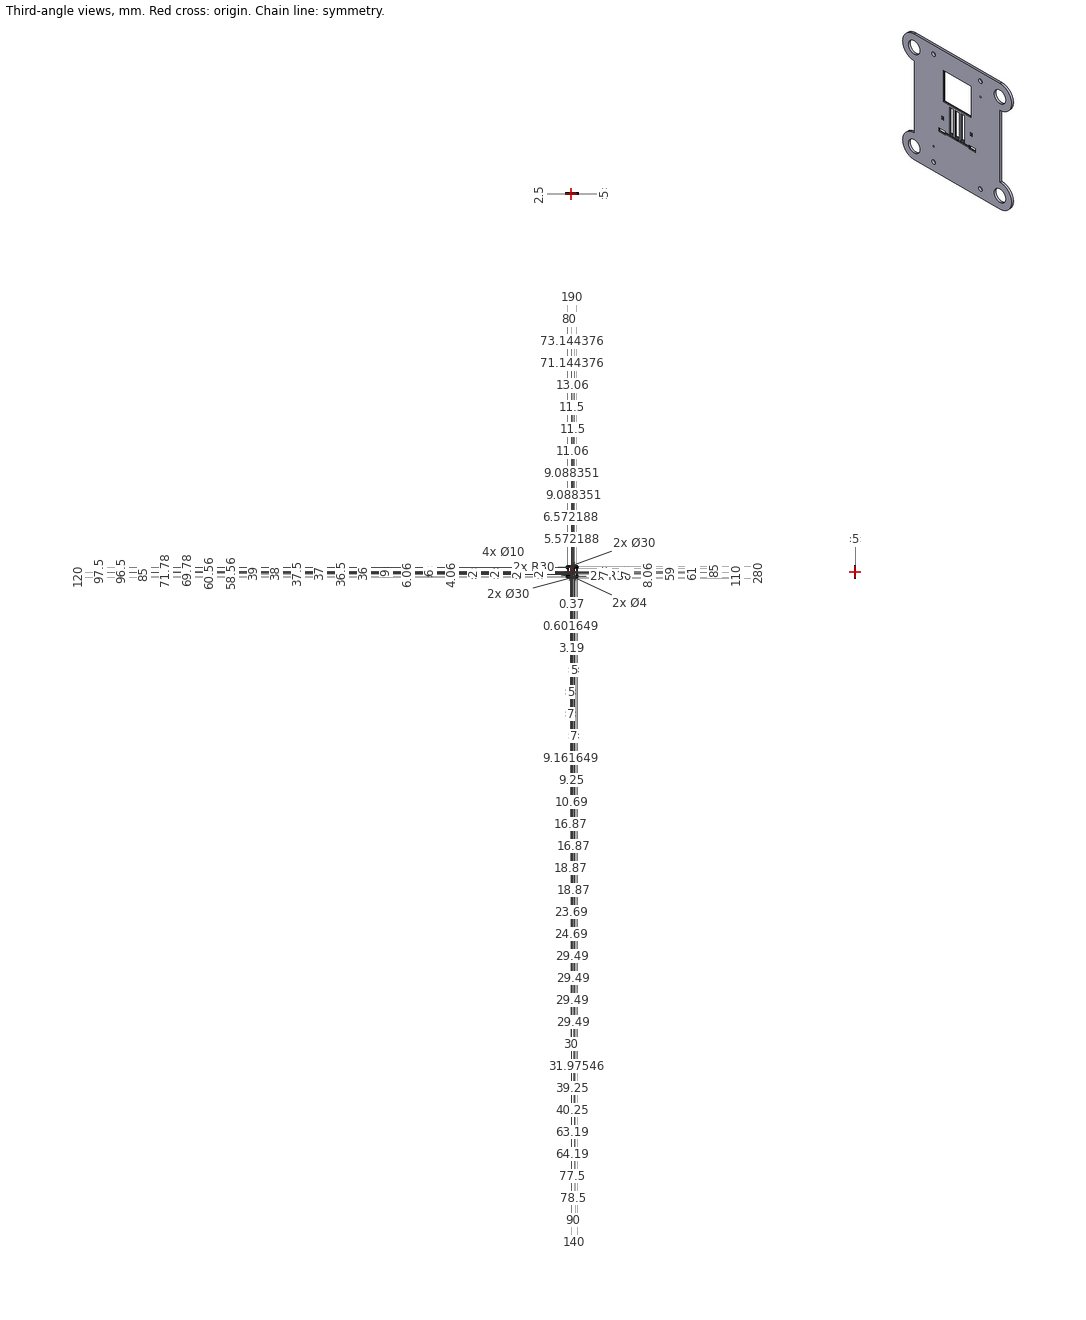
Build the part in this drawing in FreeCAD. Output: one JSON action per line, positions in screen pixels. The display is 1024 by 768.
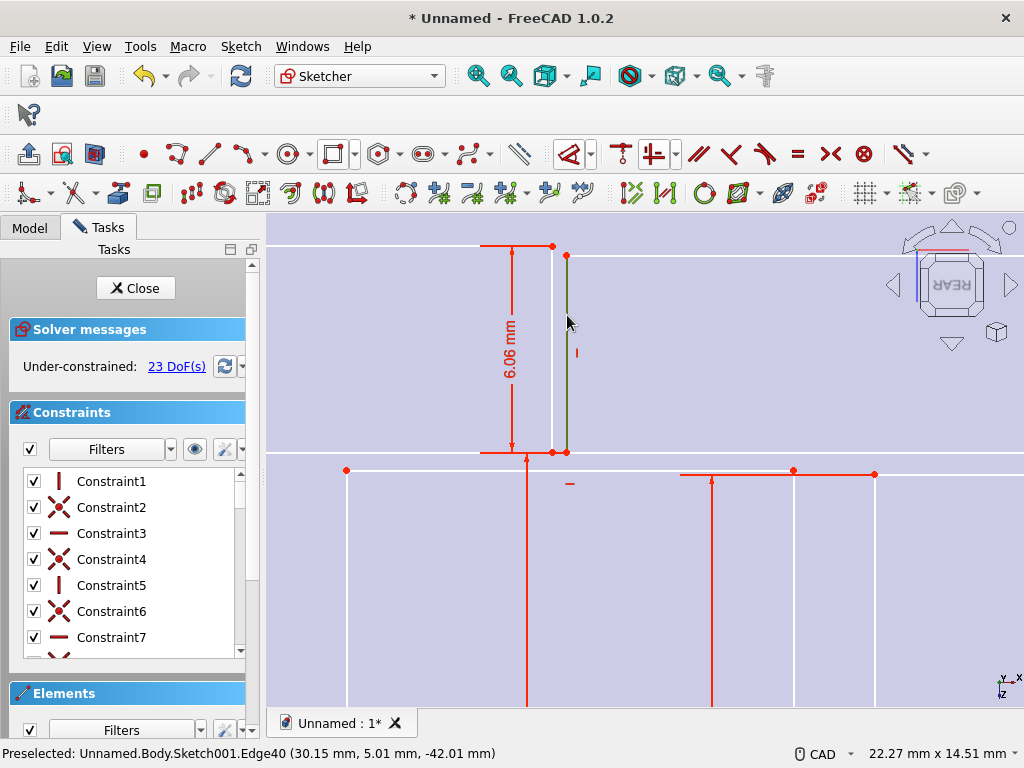
{"action": "left_click", "coordinate": [590, 154]}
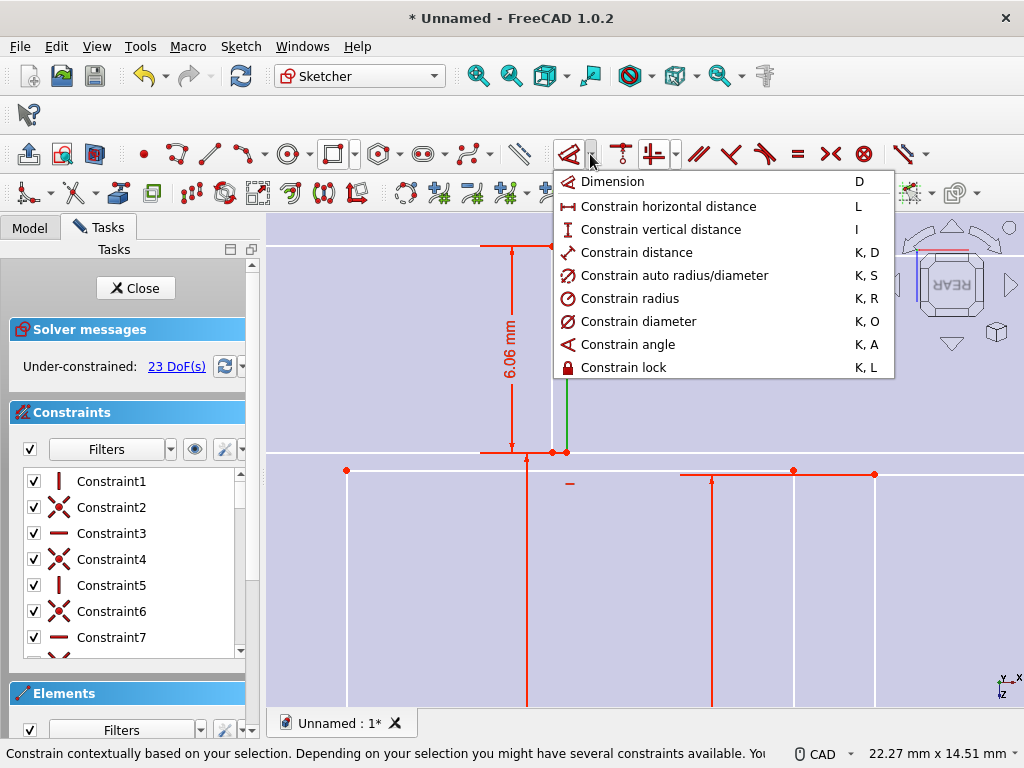
{"action": "left_click", "coordinate": [724, 230]}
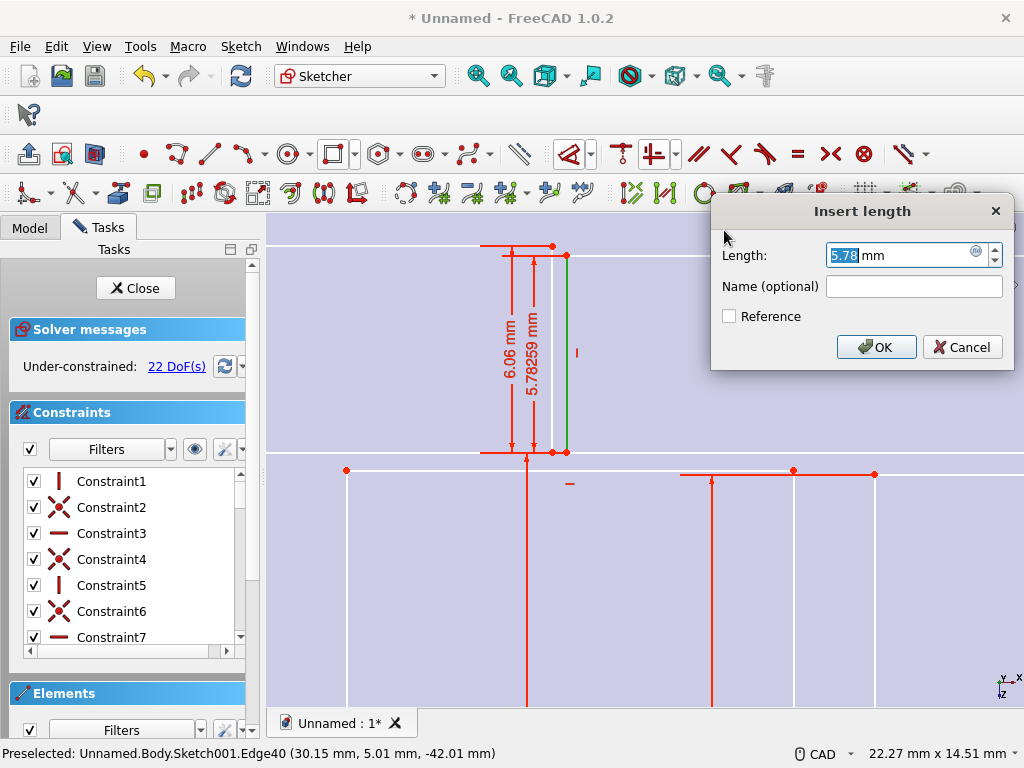
{"action": "type", "text": "6.06"}
{"action": "key", "text": "Return"}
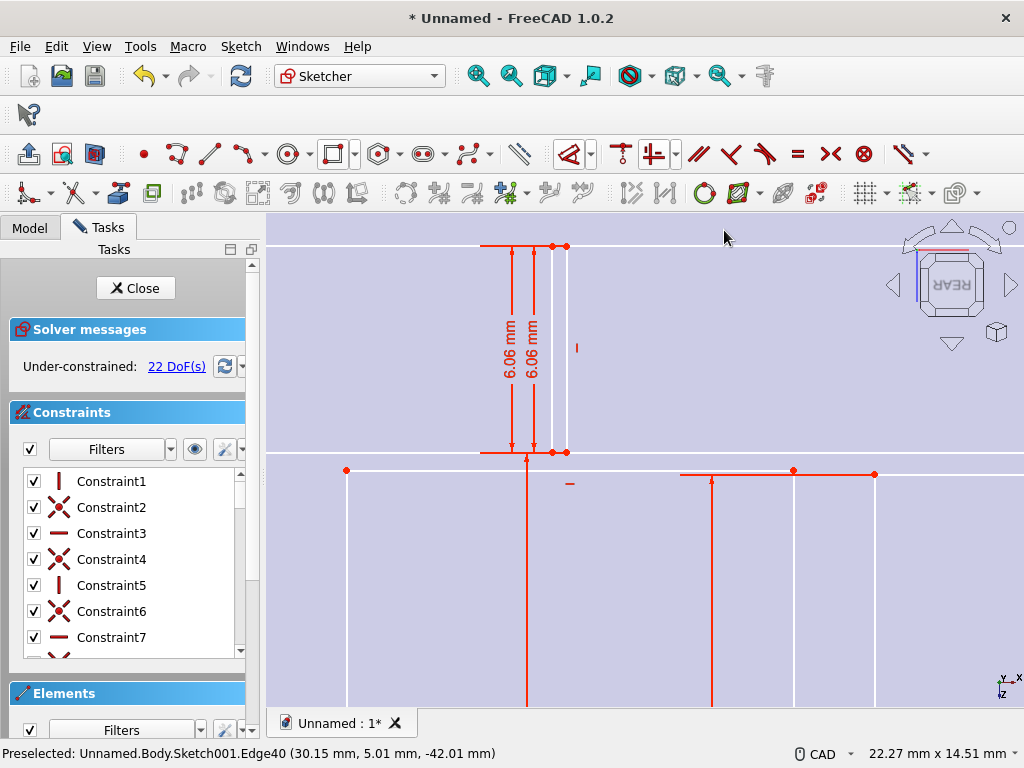
{"action": "left_click", "coordinate": [353, 452]}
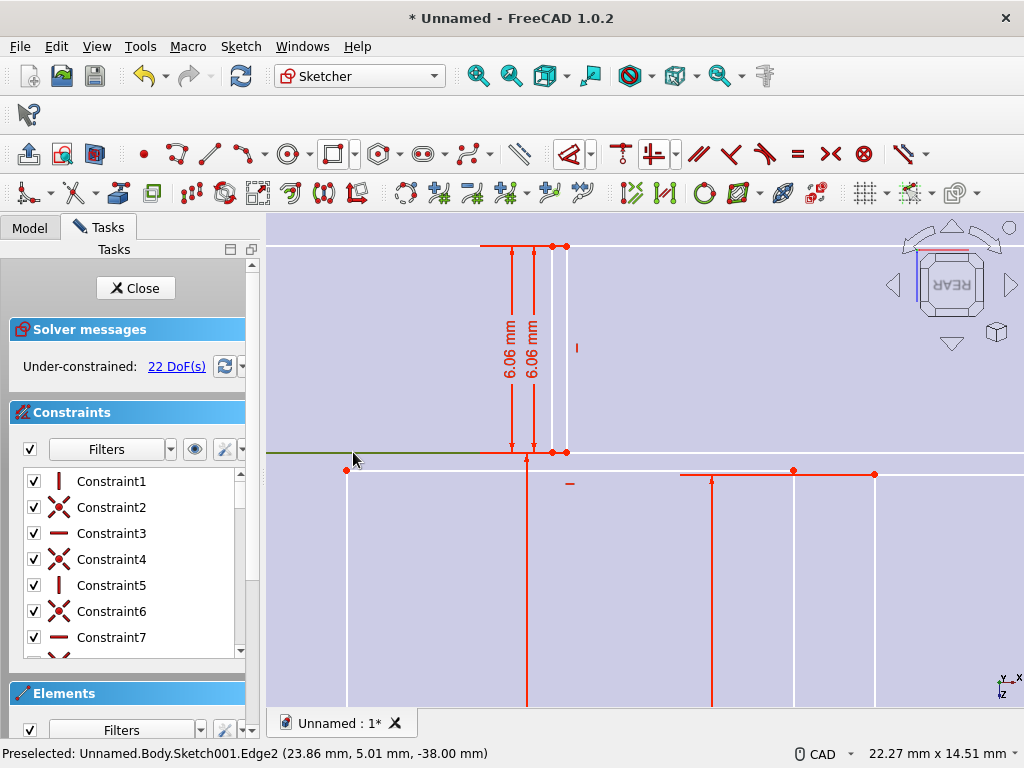
{"action": "left_click", "coordinate": [590, 154]}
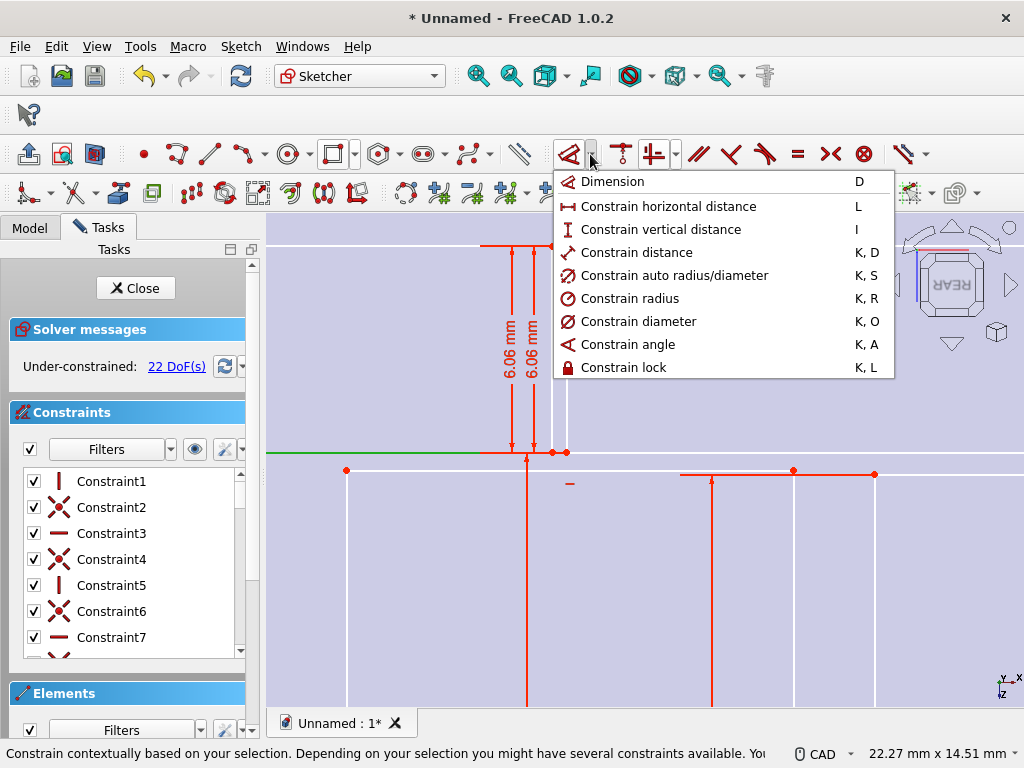
{"action": "left_click", "coordinate": [724, 206]}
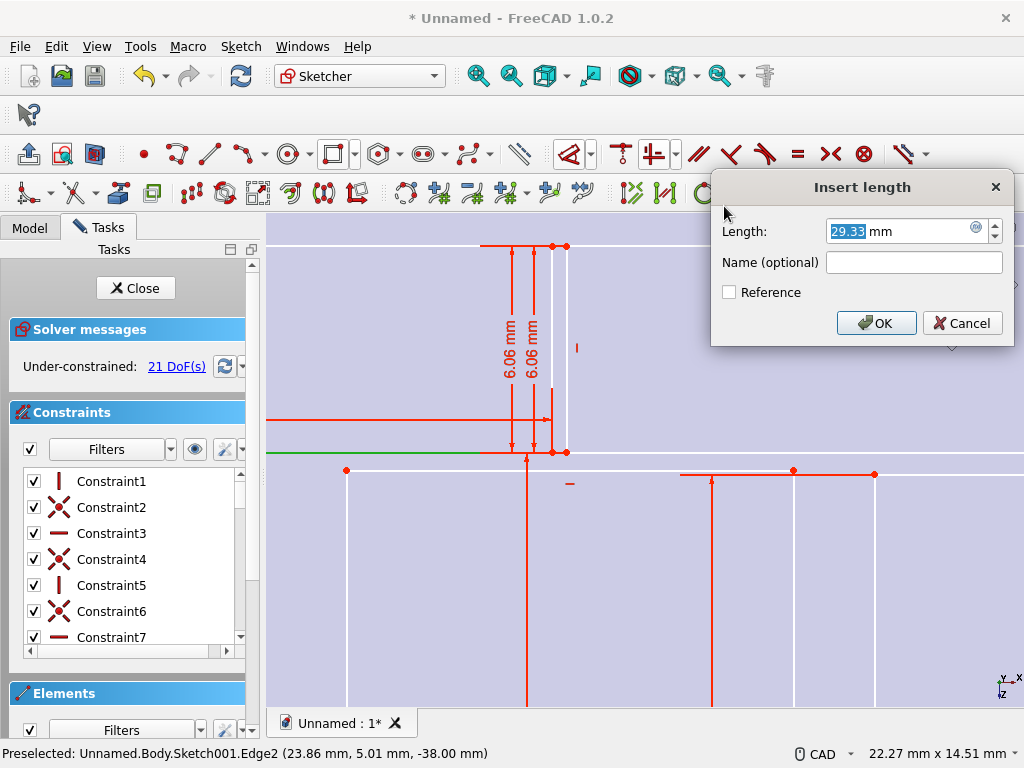
{"action": "type", "text": "29.49"}
{"action": "key", "text": "Return"}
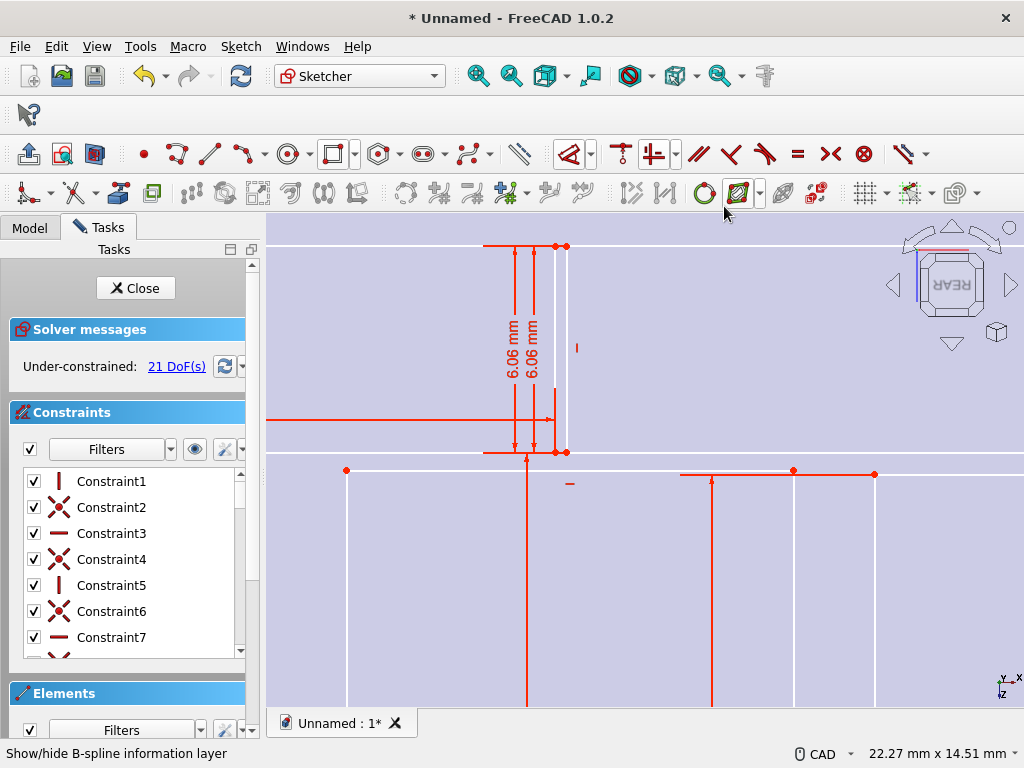
{"action": "scroll", "coordinate": [577, 320], "scroll_direction": "down", "scroll_amount": 14}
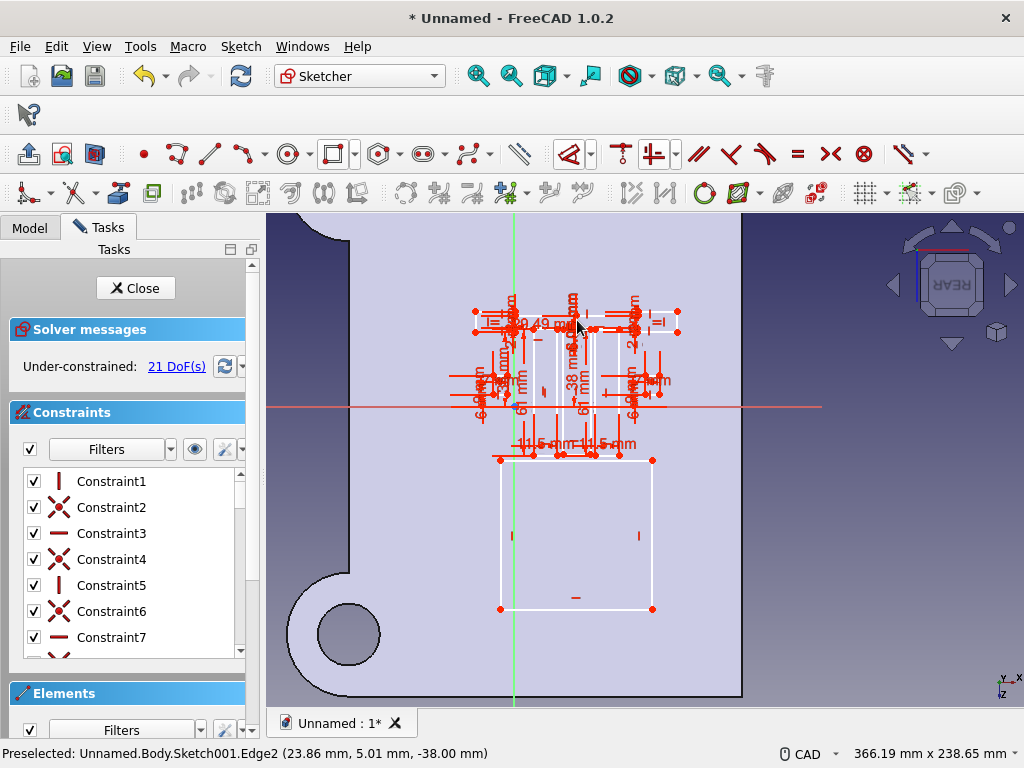
{"action": "left_click", "coordinate": [564, 316]}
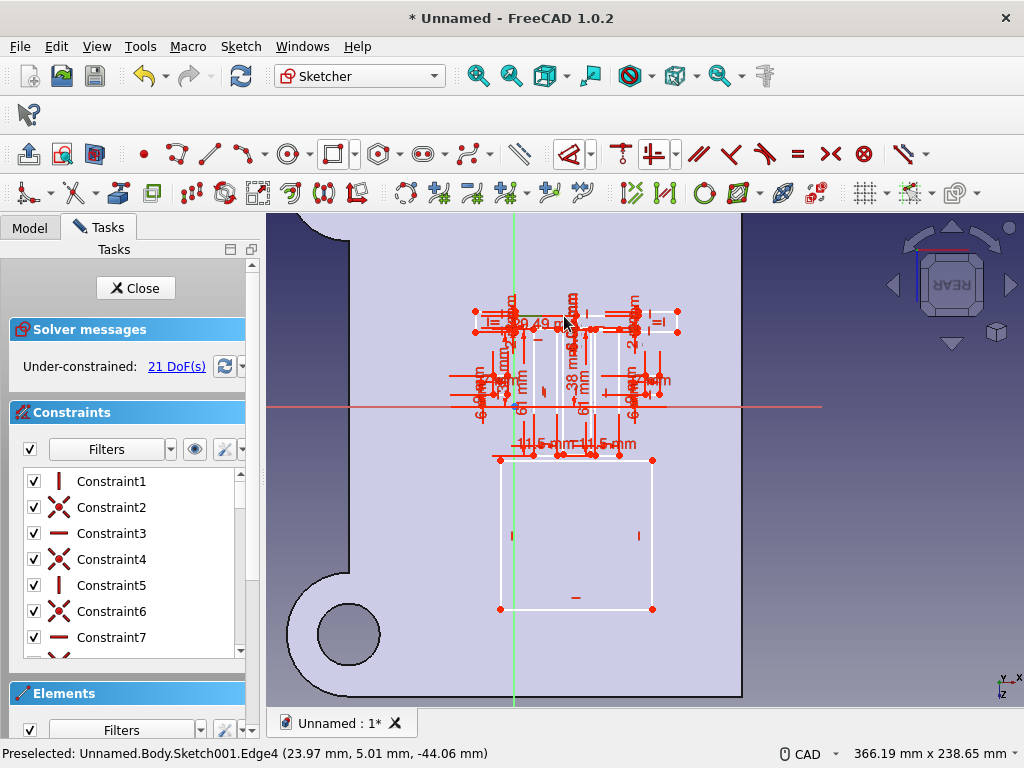
{"action": "key", "text": "l"}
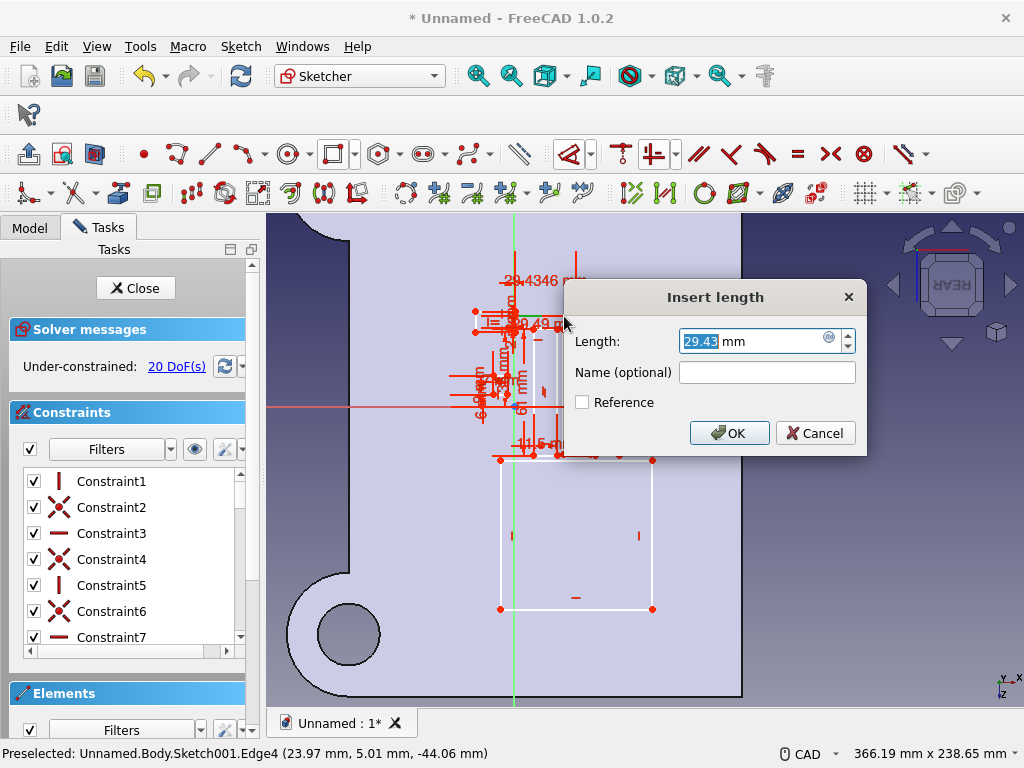
{"action": "type", "text": "29.49"}
{"action": "key", "text": "Return"}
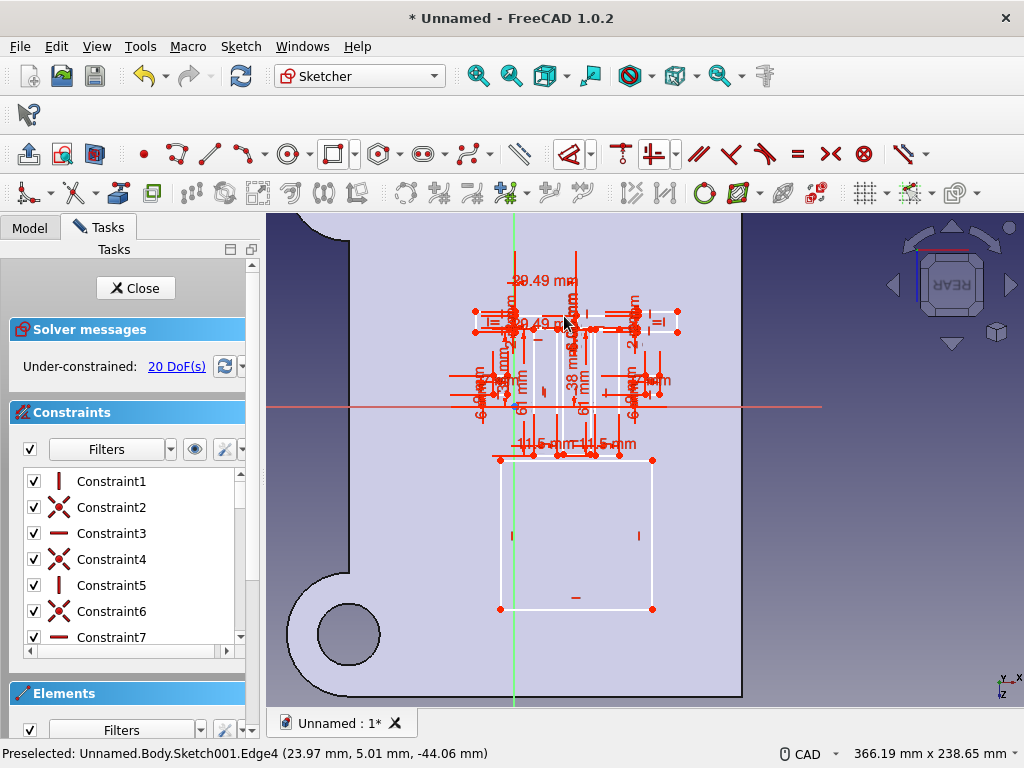
{"action": "scroll", "coordinate": [503, 312], "scroll_direction": "up", "scroll_amount": 2}